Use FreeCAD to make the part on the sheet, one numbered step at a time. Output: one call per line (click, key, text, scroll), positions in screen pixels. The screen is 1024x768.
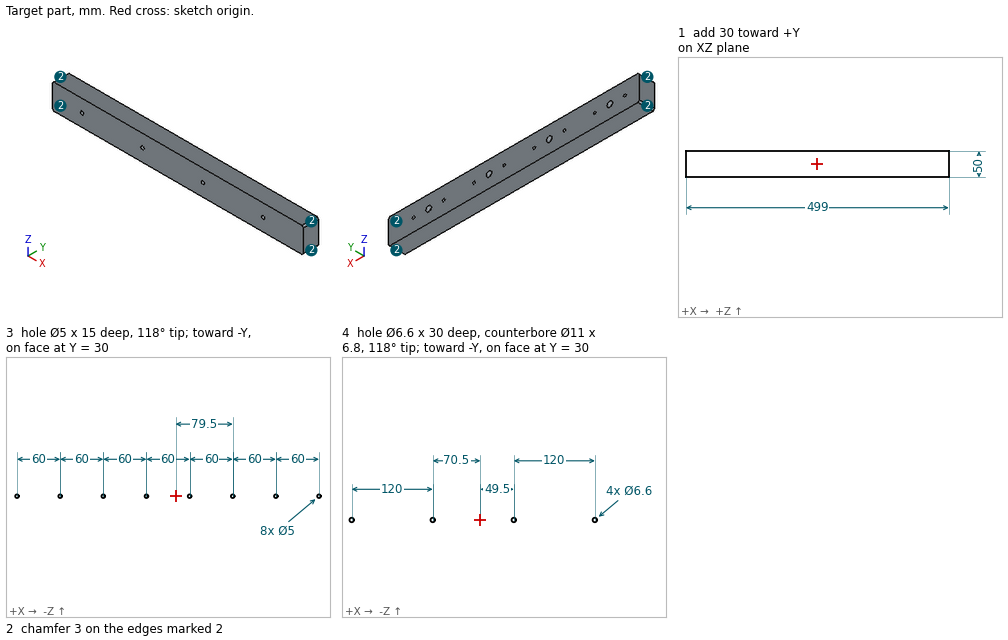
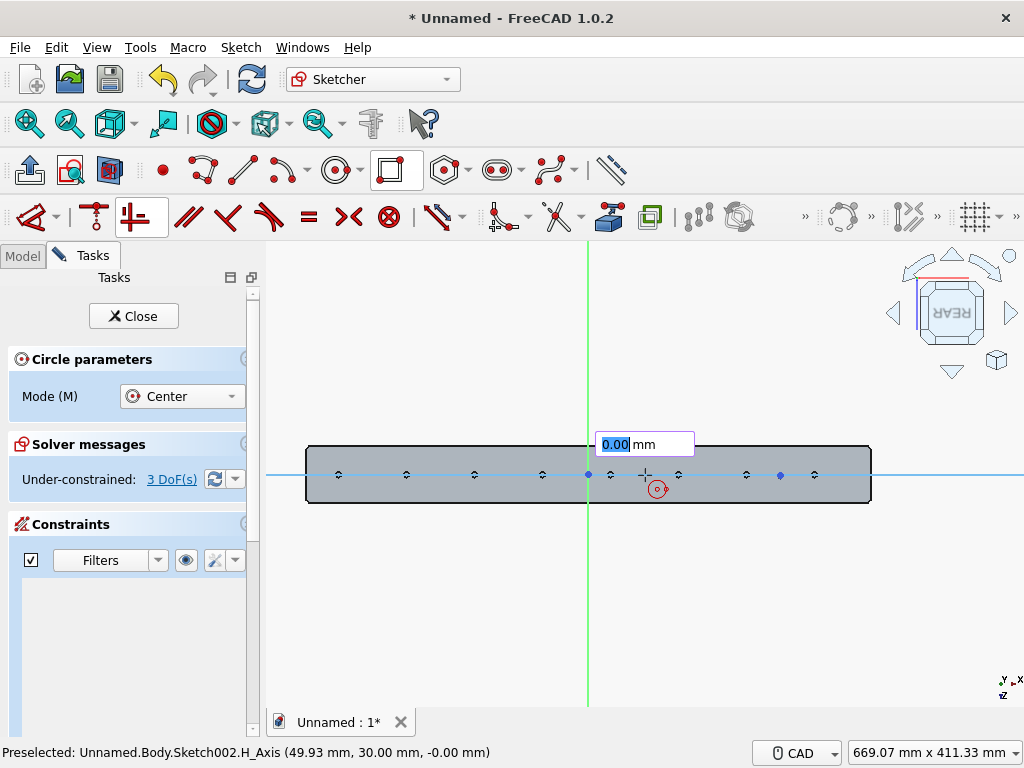
scroll(643, 478, up, 8)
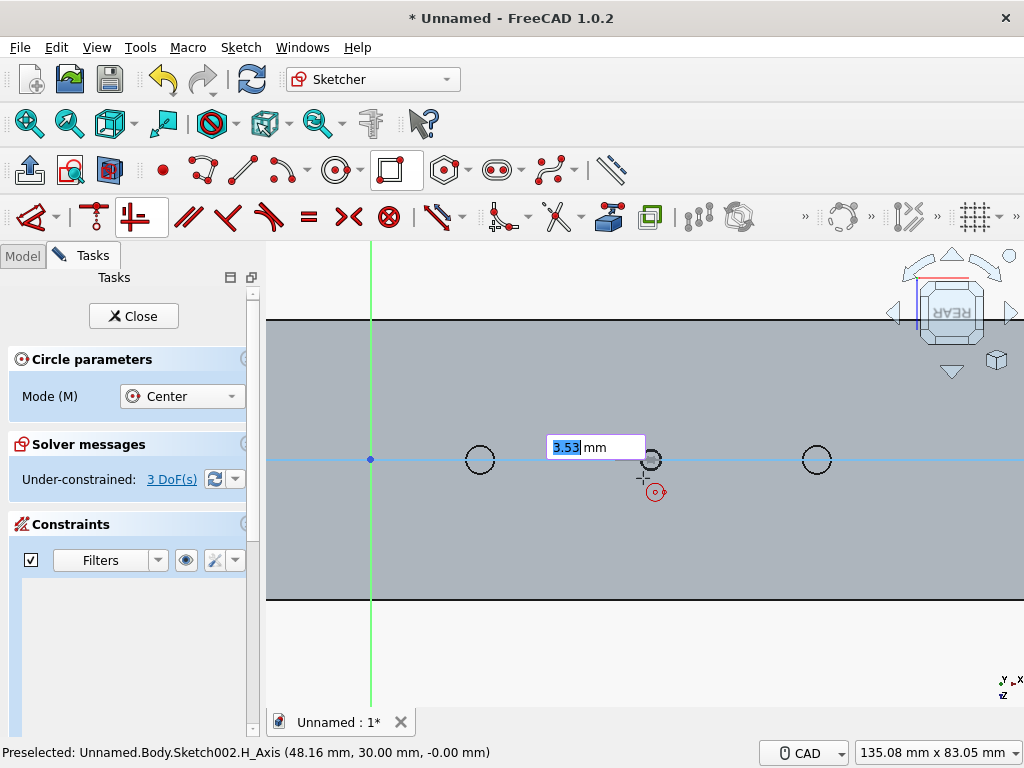
click(642, 477)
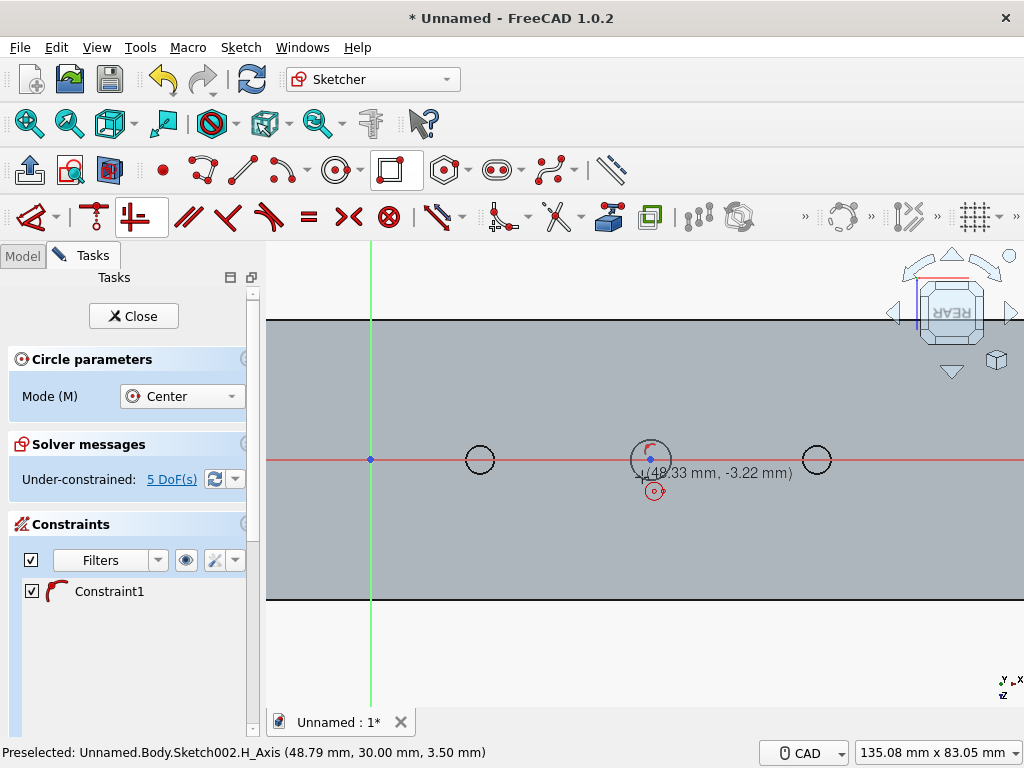
scroll(643, 478, down, 8)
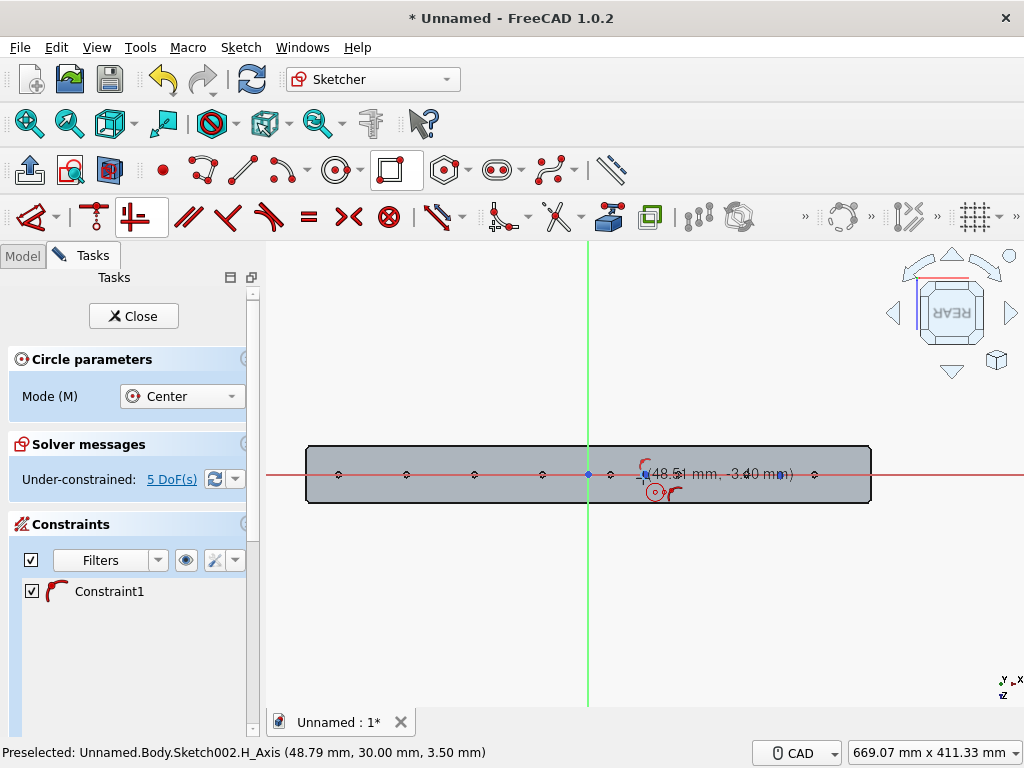
scroll(509, 475, up, 10)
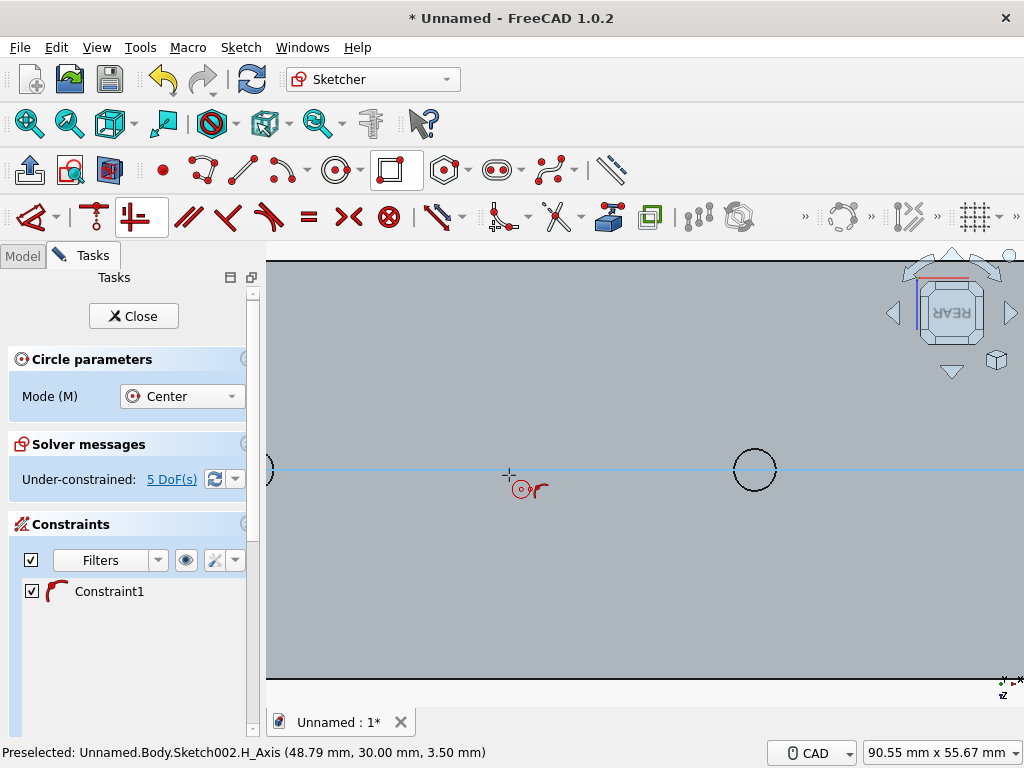
scroll(509, 475, down, 10)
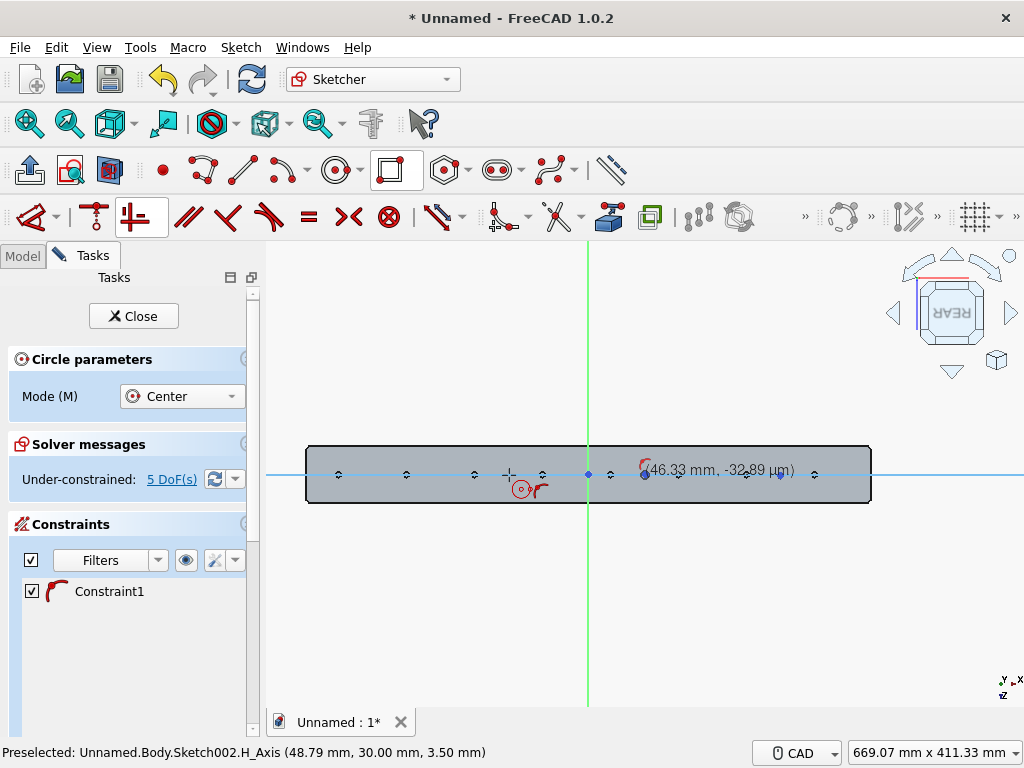
click(509, 475)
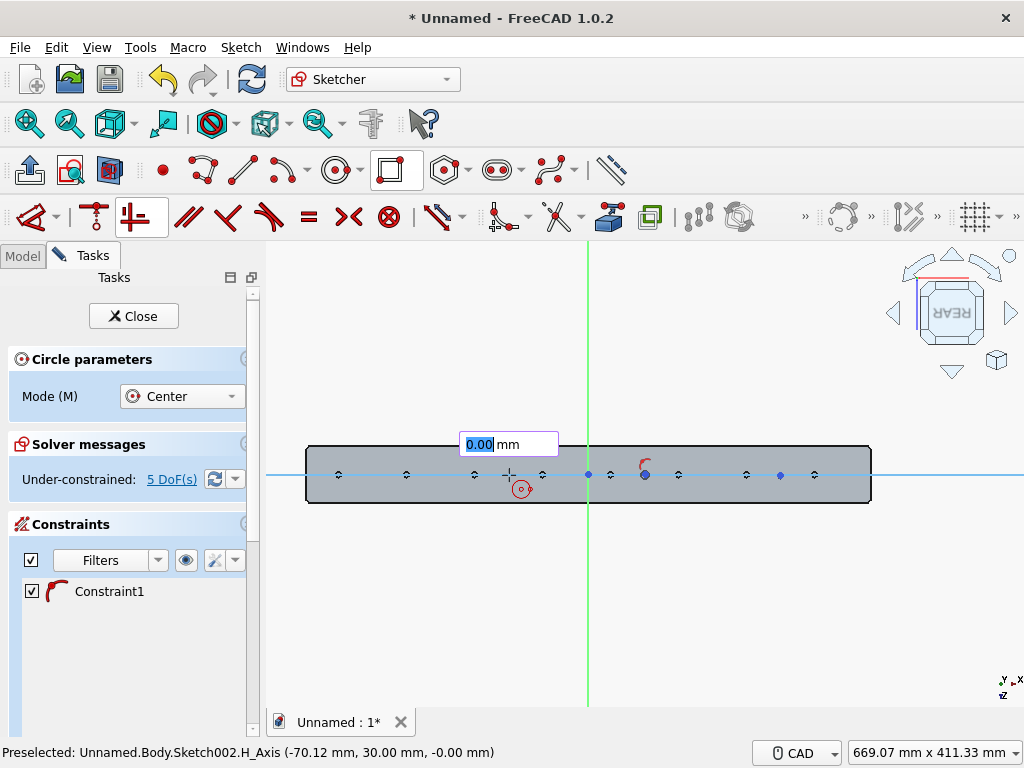
scroll(507, 478, up, 8)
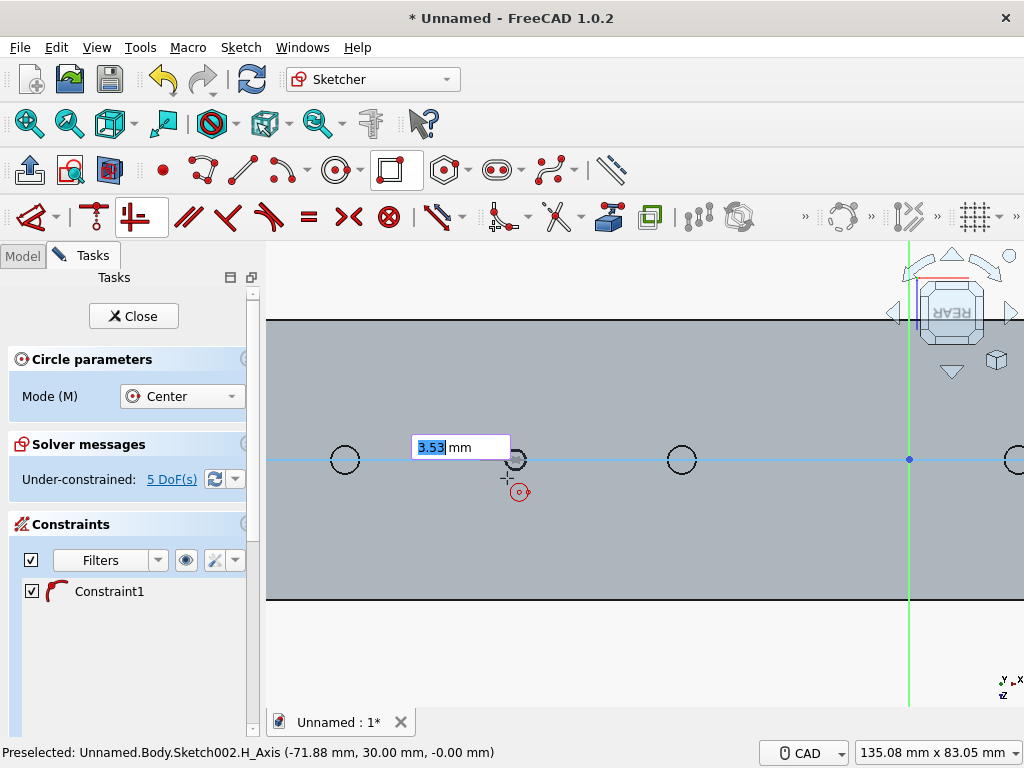
click(507, 477)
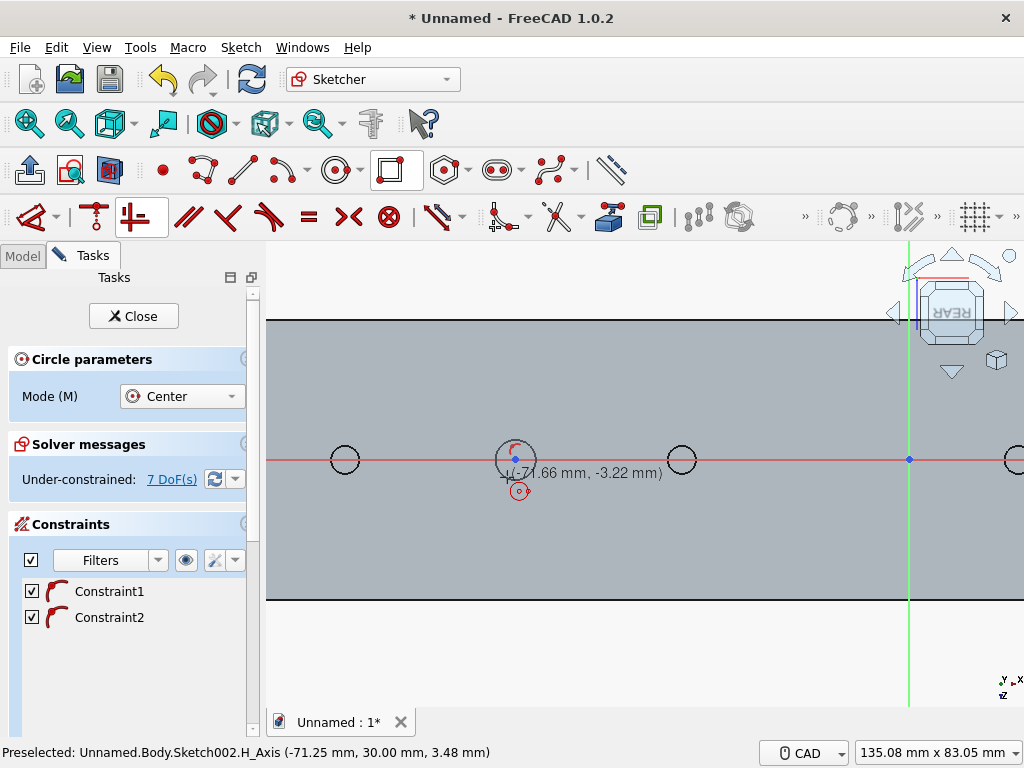
scroll(507, 478, down, 8)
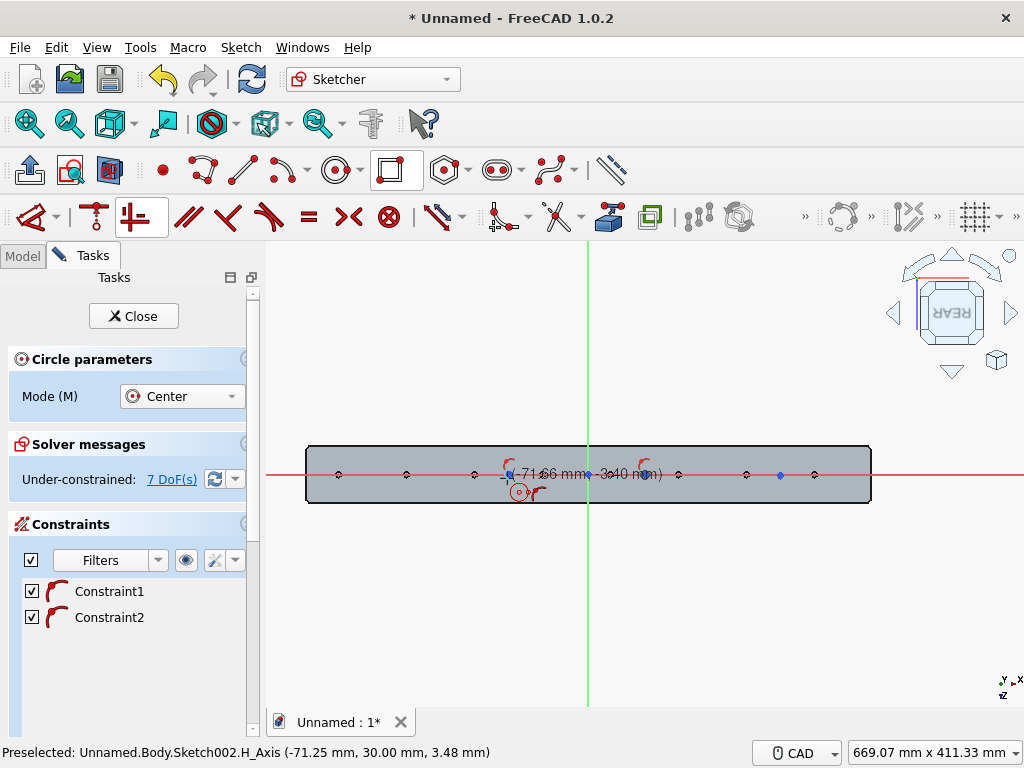
scroll(373, 475, up, 10)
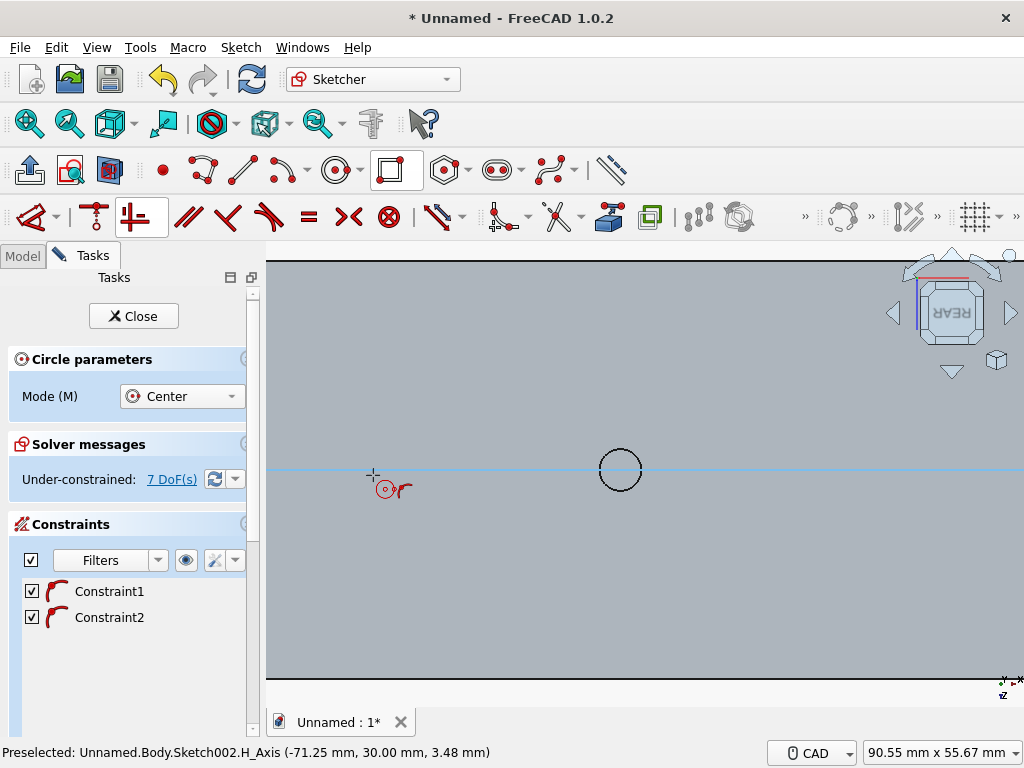
scroll(373, 475, down, 10)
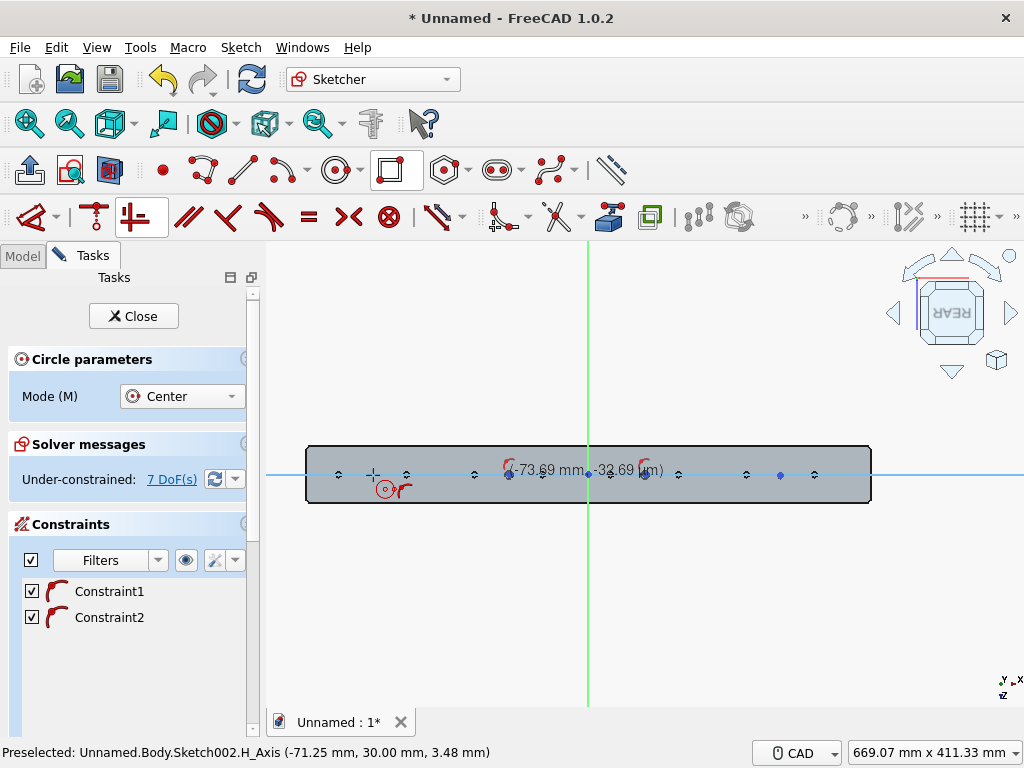
click(373, 475)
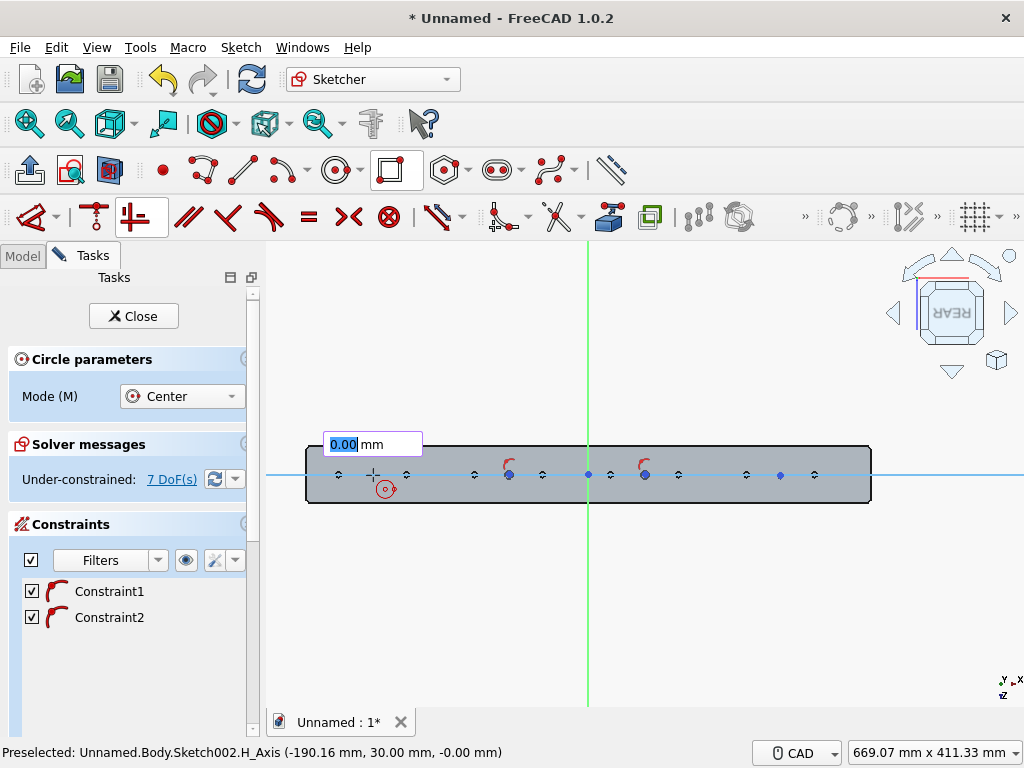
scroll(371, 478, up, 8)